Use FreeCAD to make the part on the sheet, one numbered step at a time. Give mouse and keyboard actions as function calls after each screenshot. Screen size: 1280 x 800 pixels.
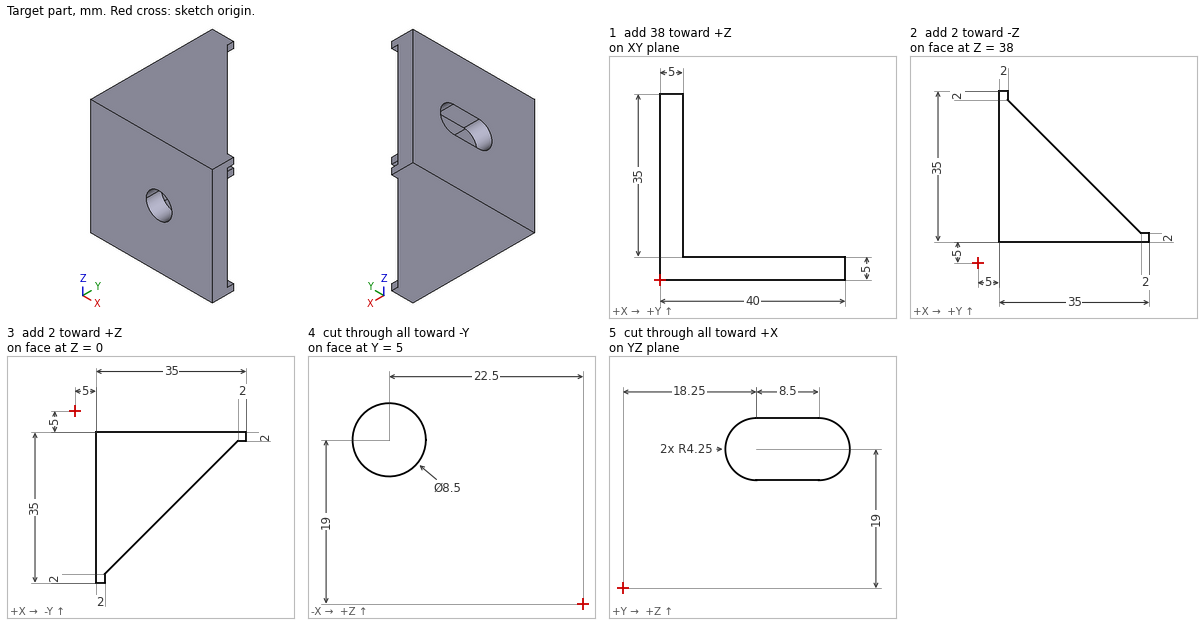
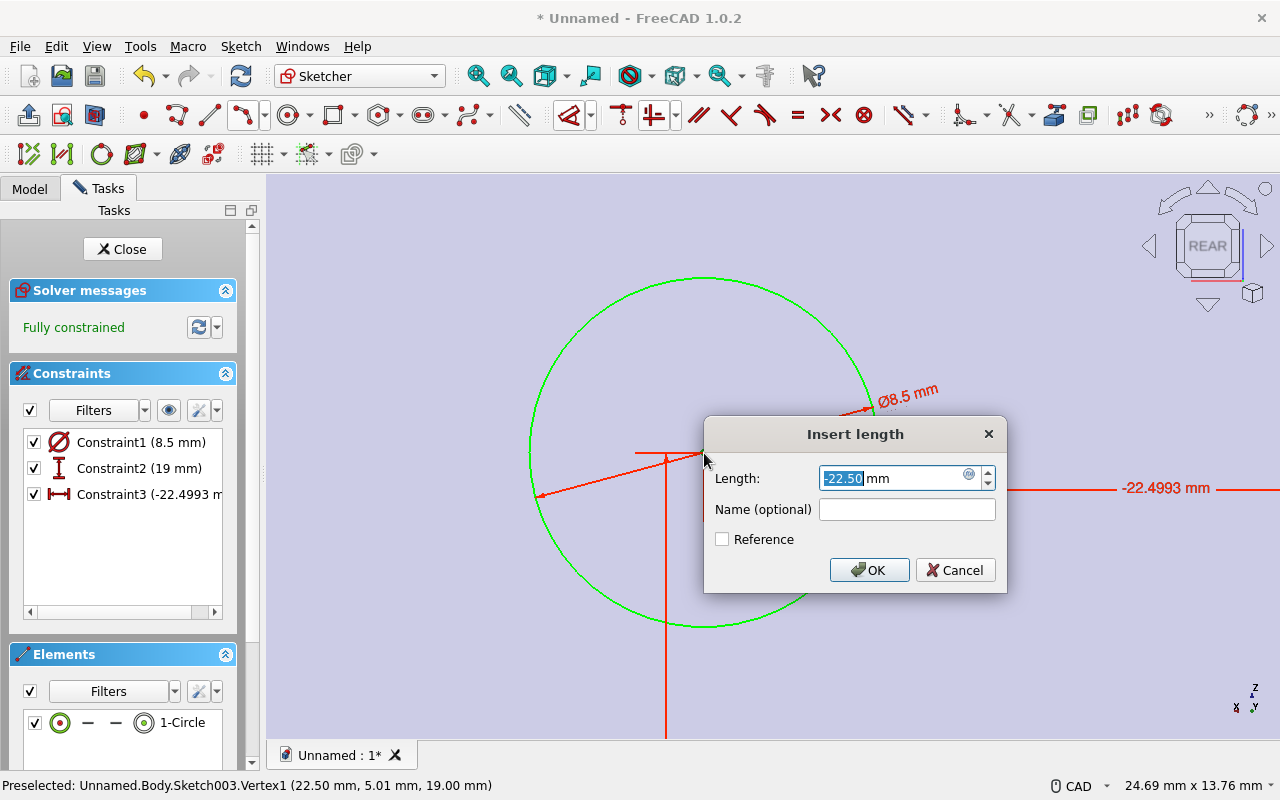
text(-22.5)
key(Return)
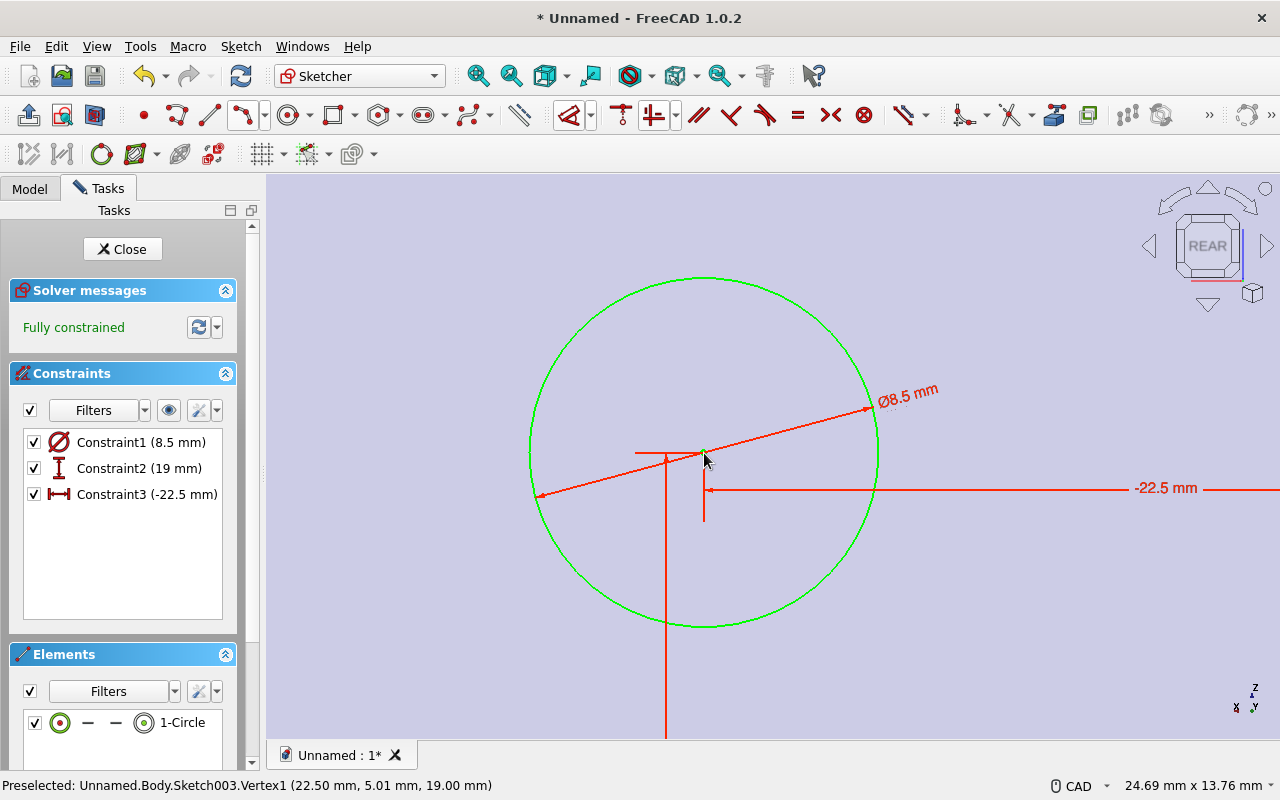
click(123, 249)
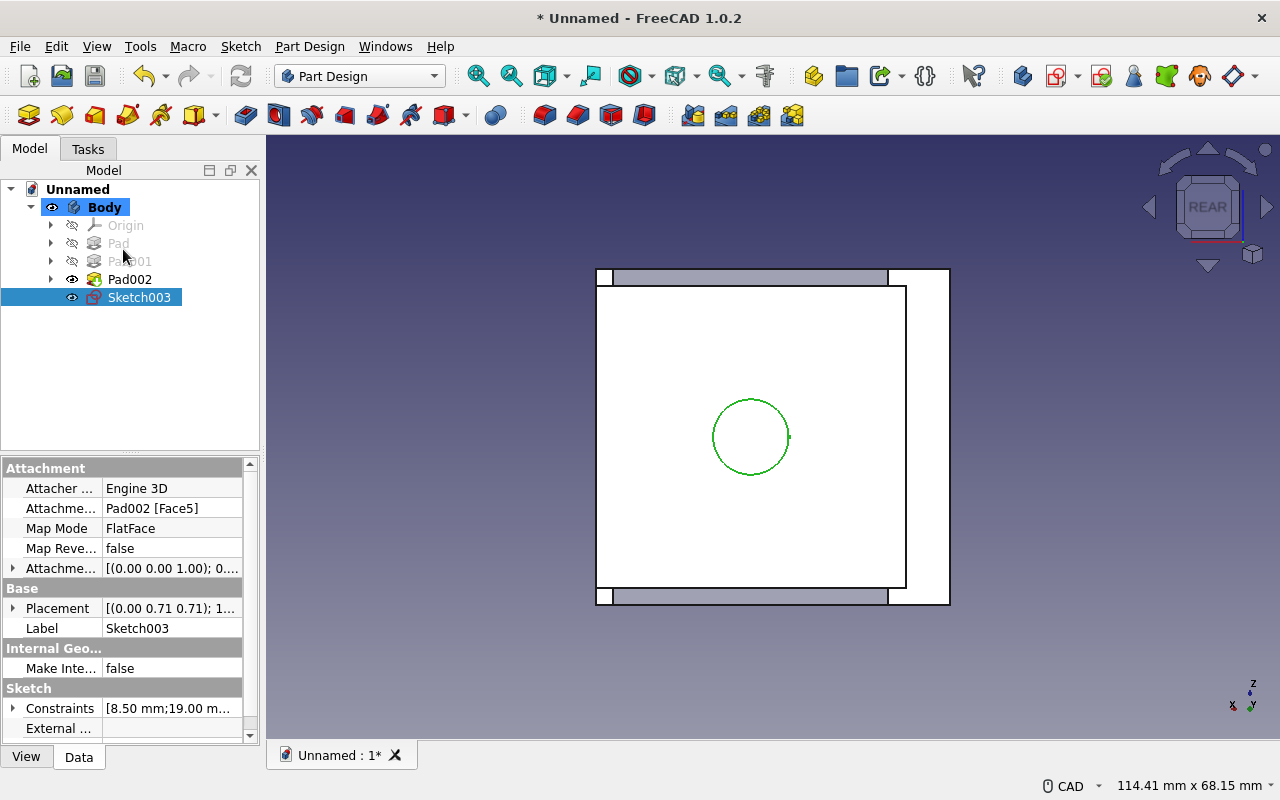
click(246, 116)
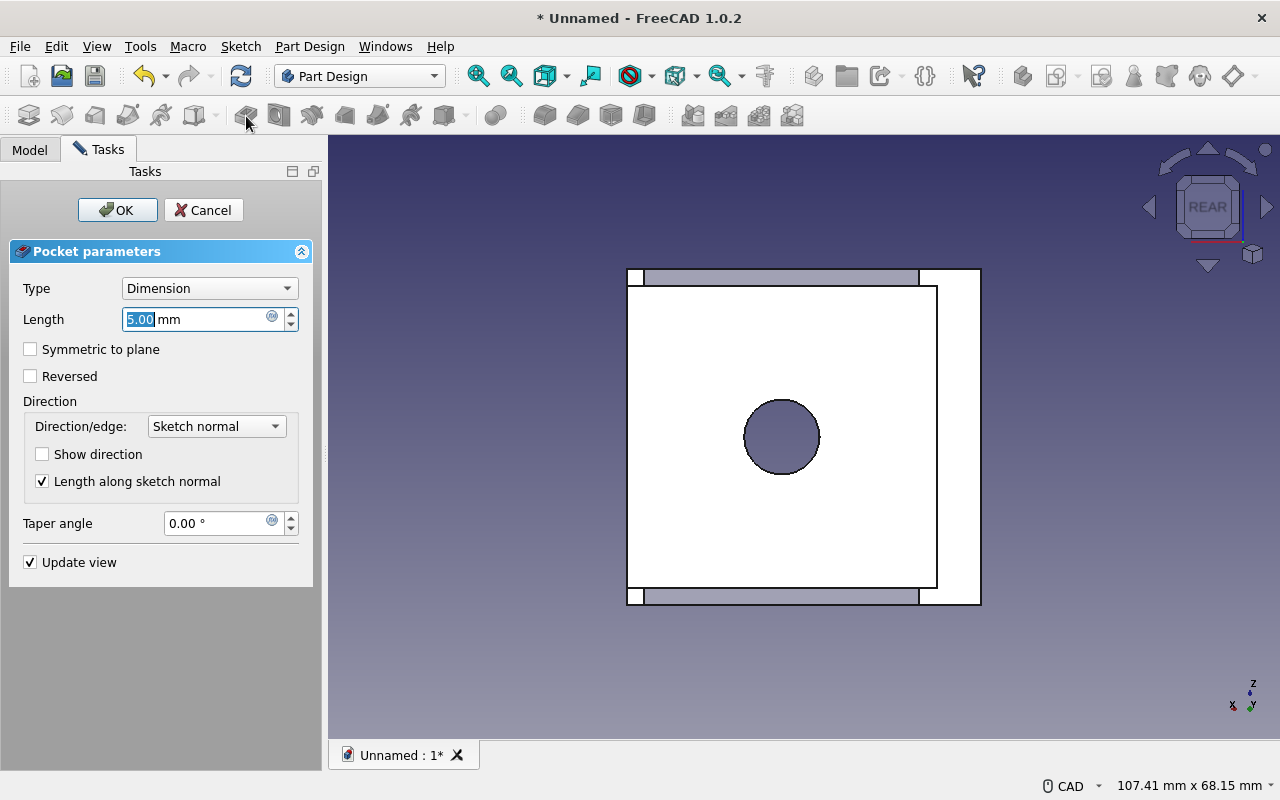
click(210, 288)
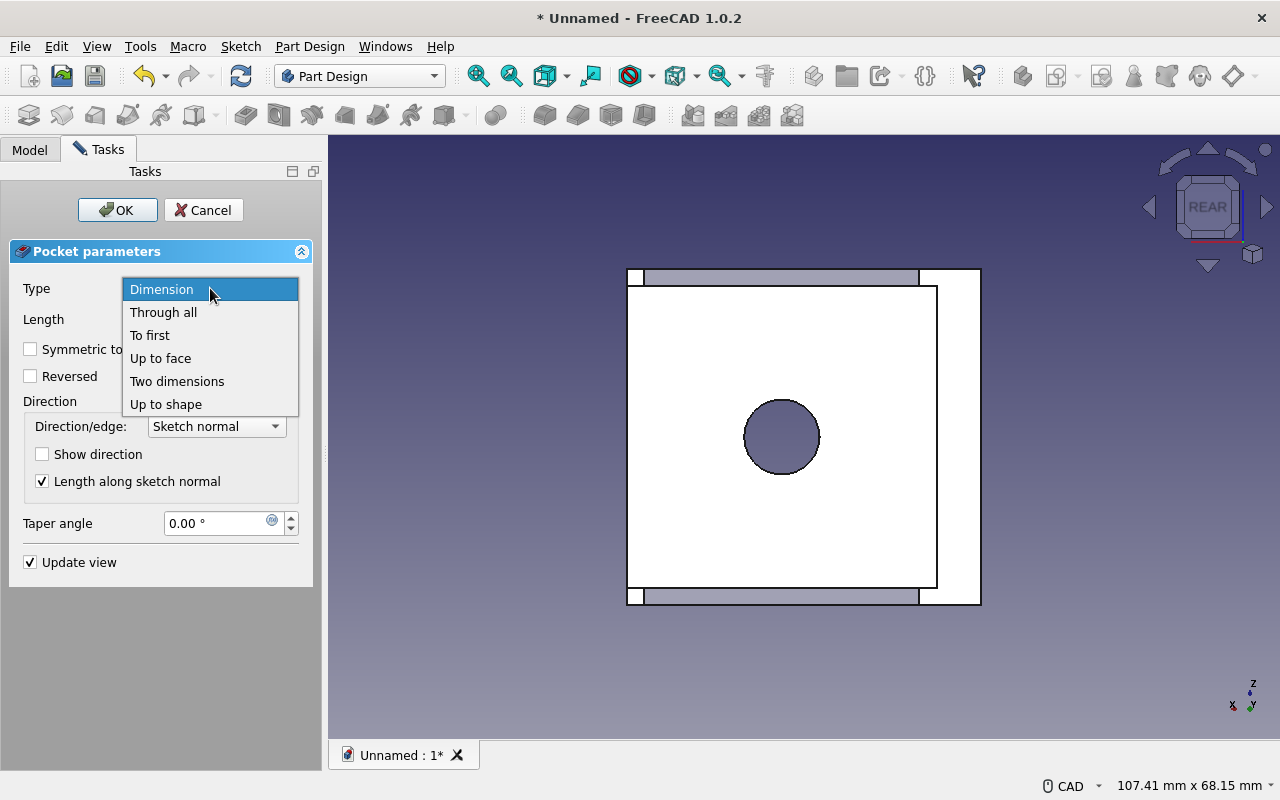
click(208, 312)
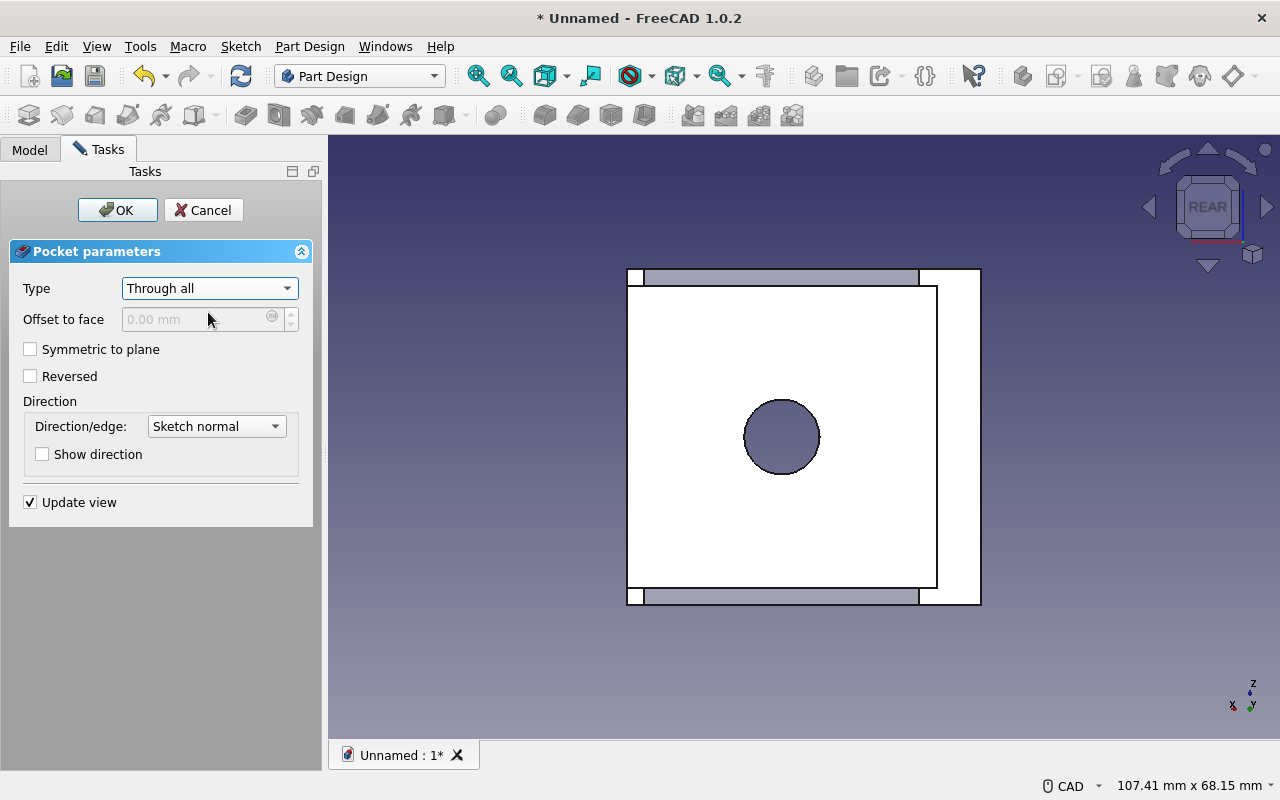
click(118, 210)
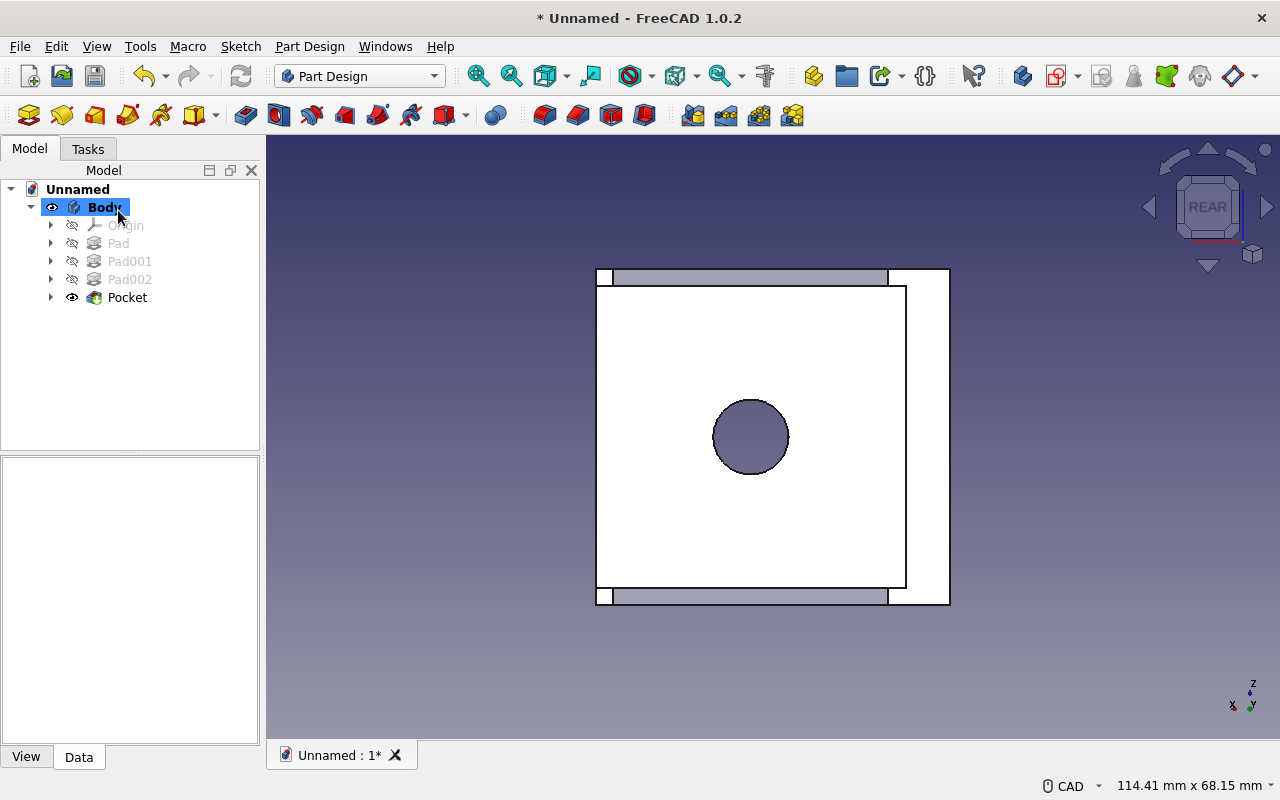
click(1056, 76)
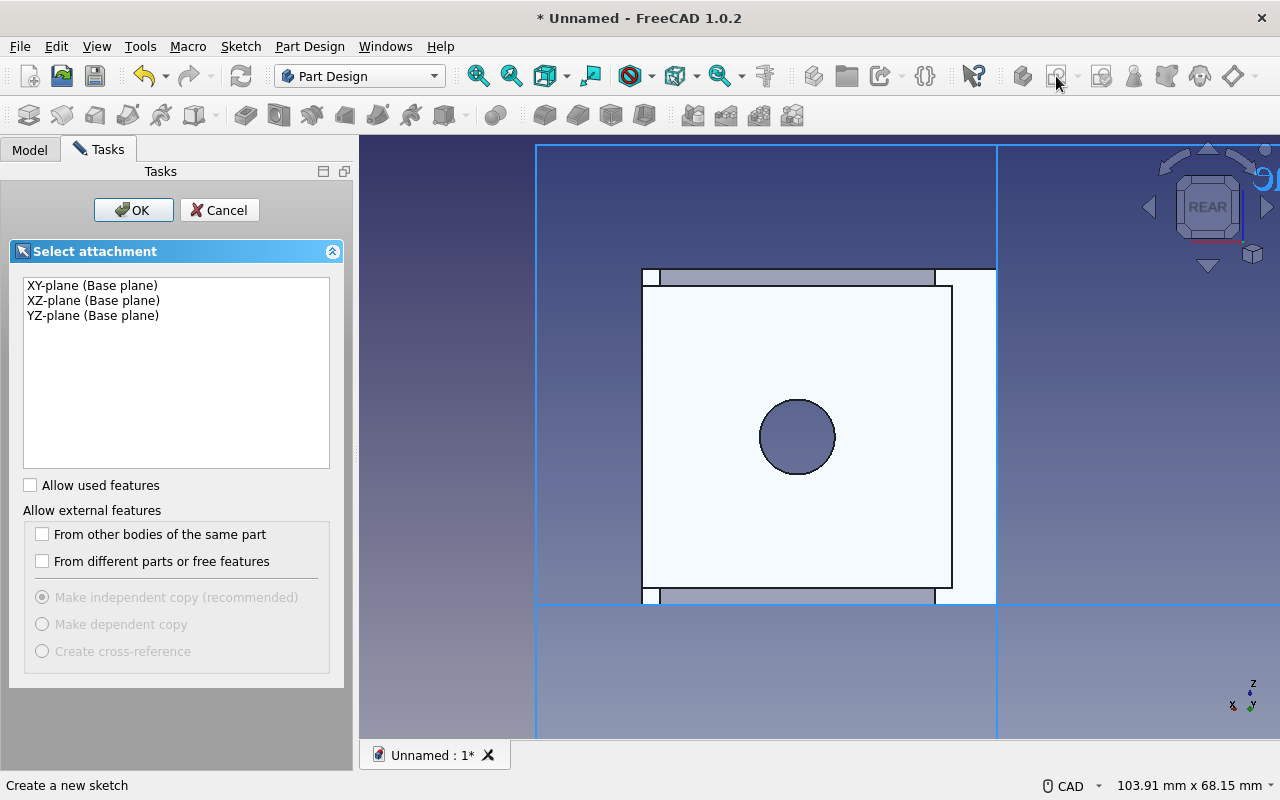
click(84, 316)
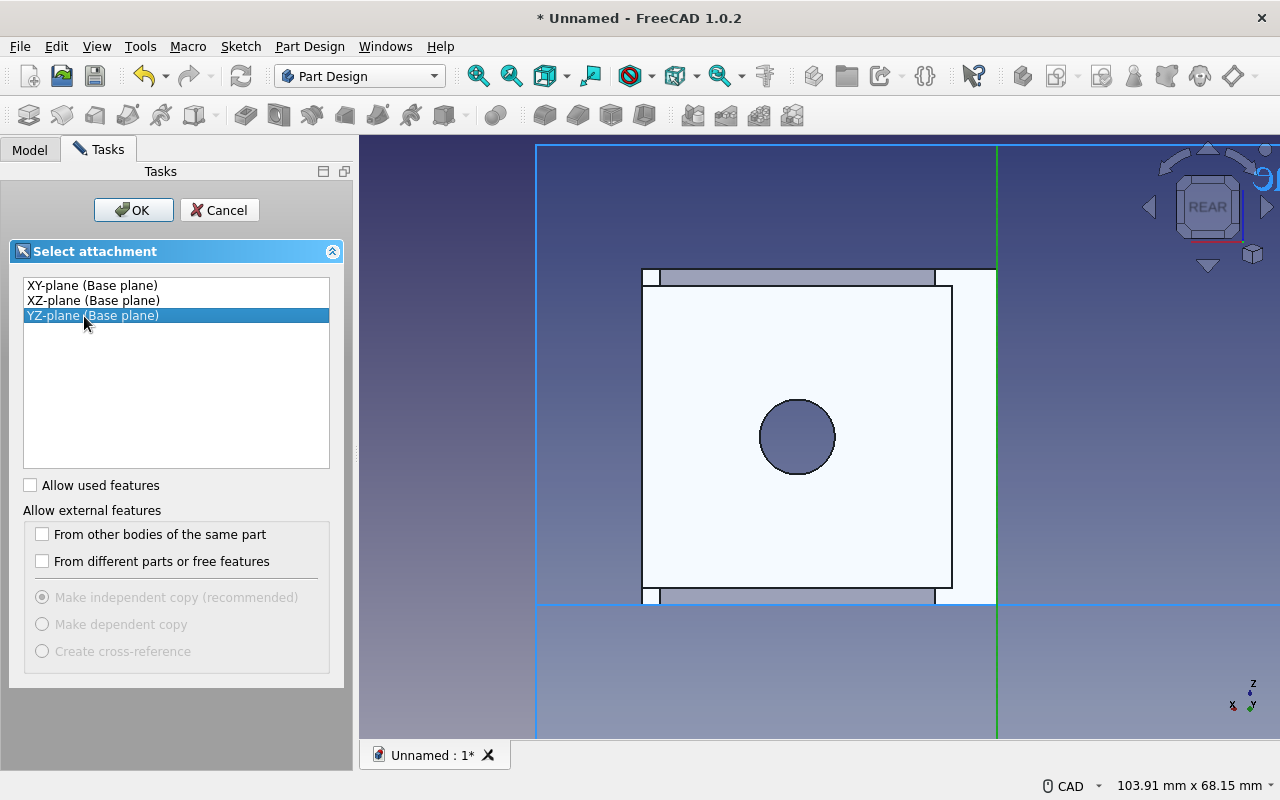
click(134, 210)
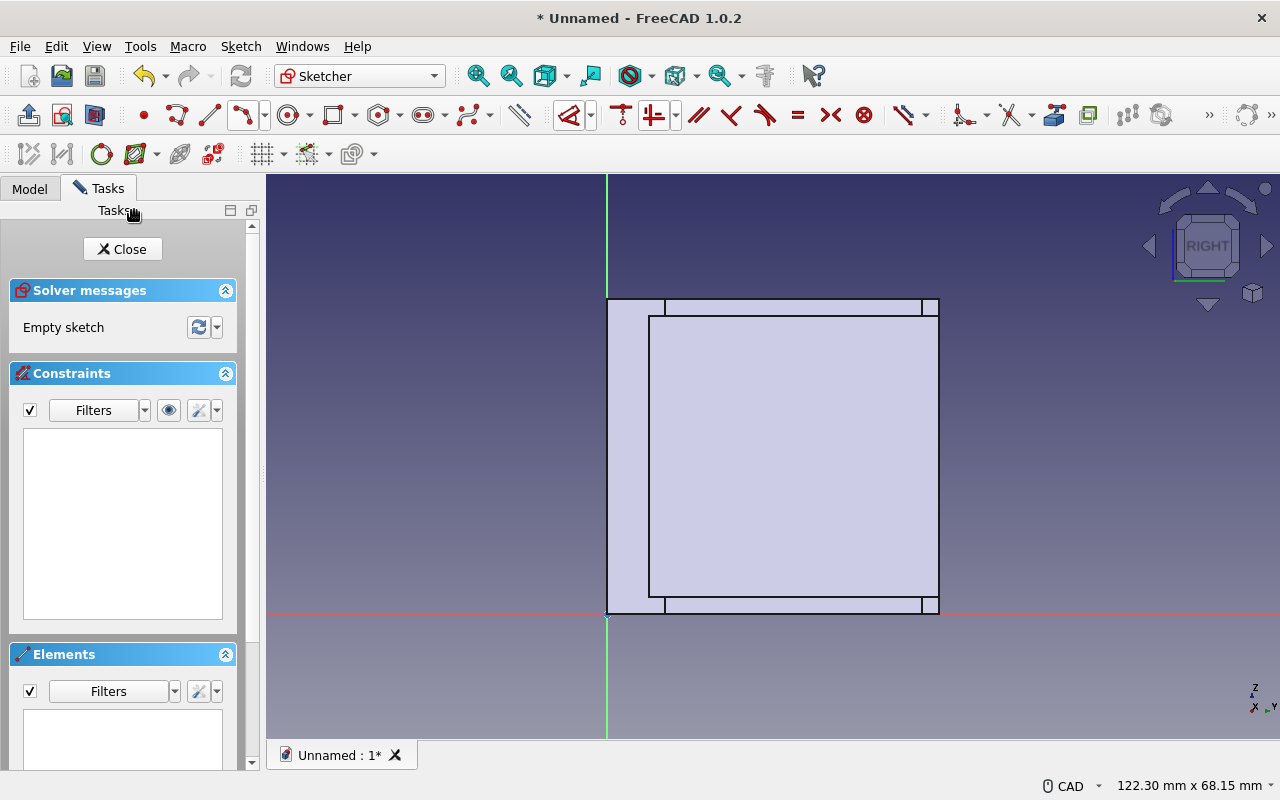
key(q)
key(s)